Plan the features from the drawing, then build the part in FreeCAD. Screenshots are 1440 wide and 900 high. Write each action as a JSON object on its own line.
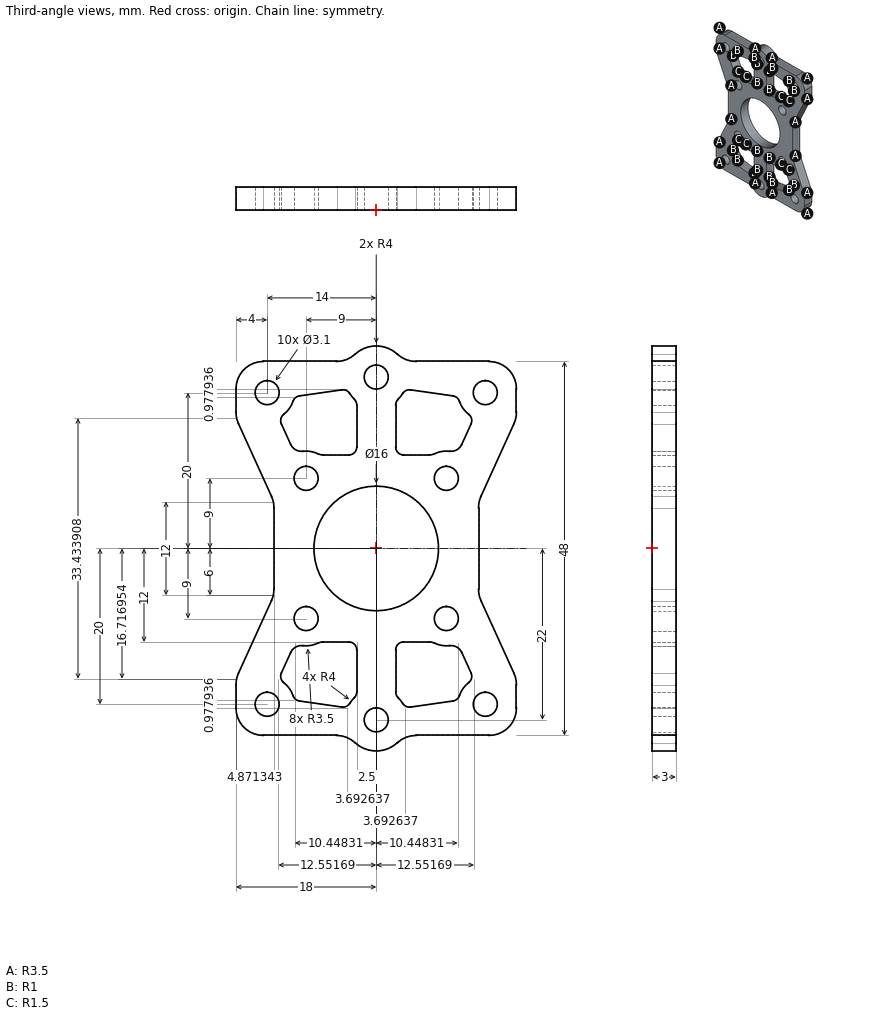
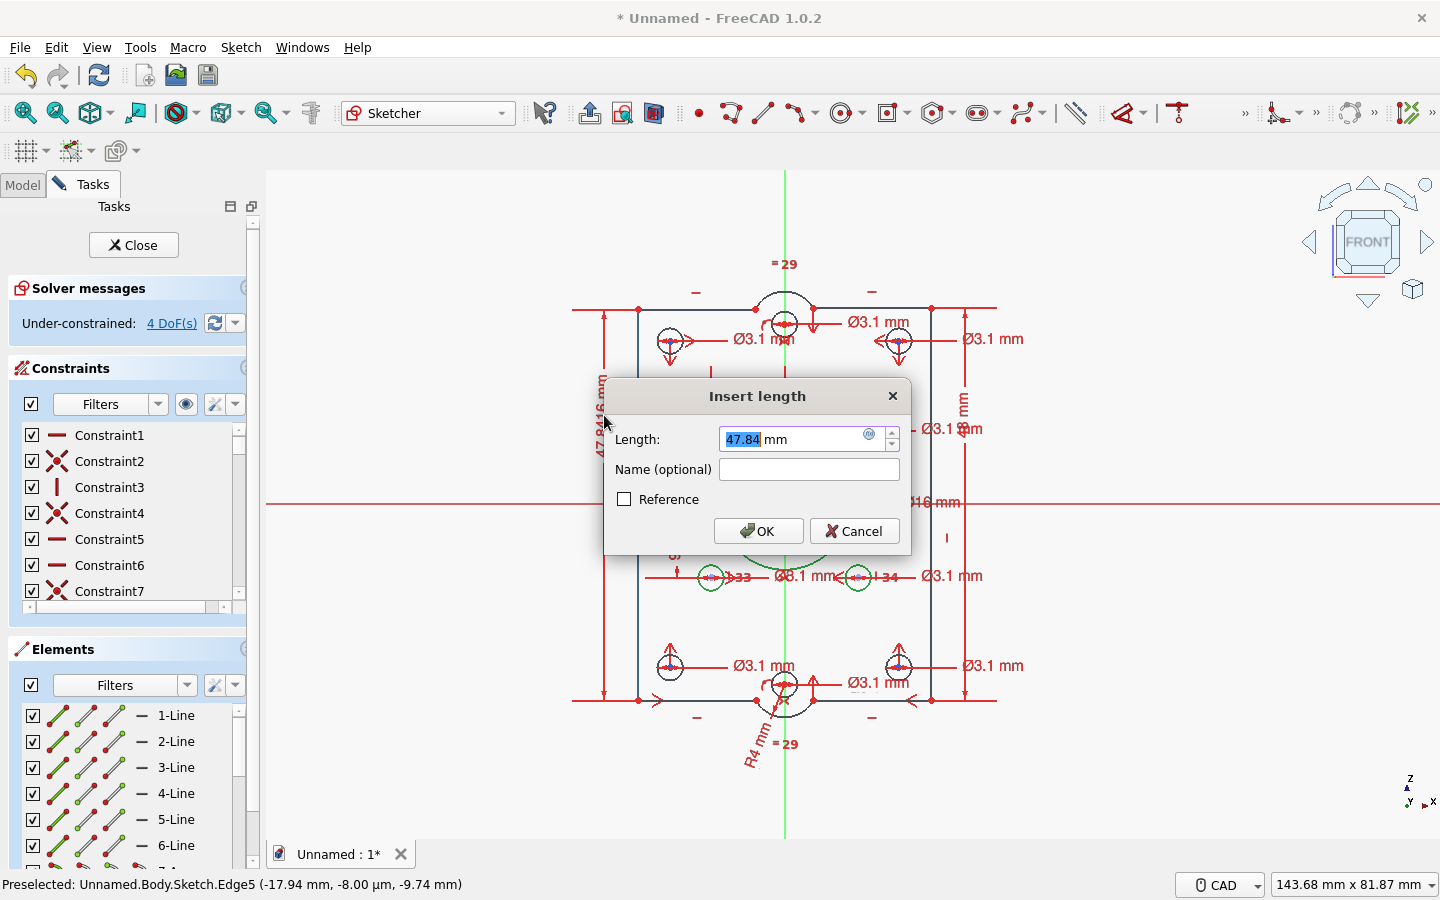
{"action": "type", "text": "48"}
{"action": "key", "text": "Return"}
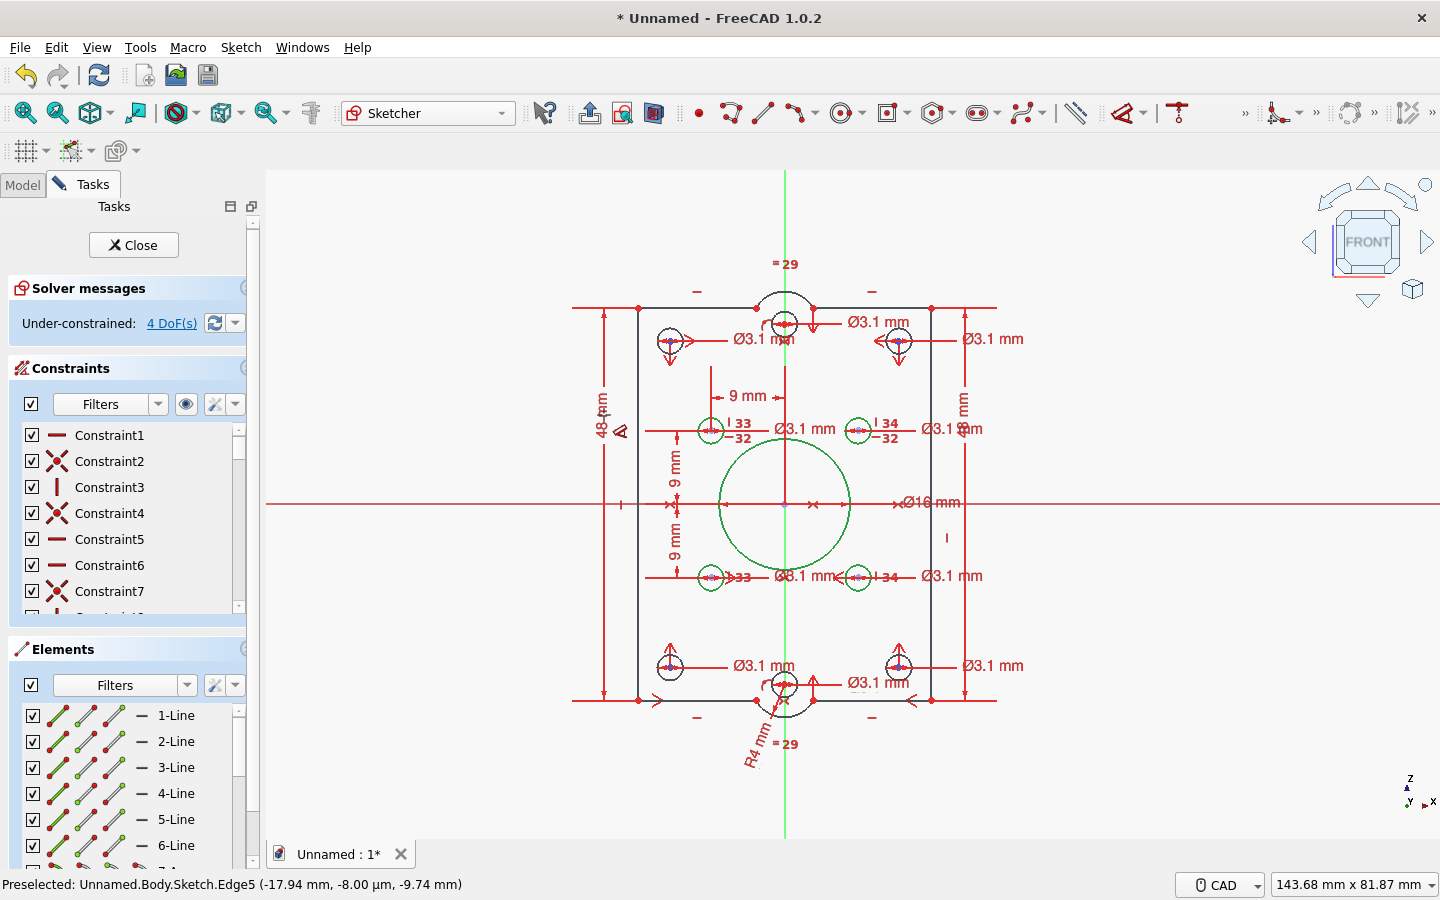
{"action": "left_click", "coordinate": [670, 341]}
{"action": "left_click", "coordinate": [754, 538]}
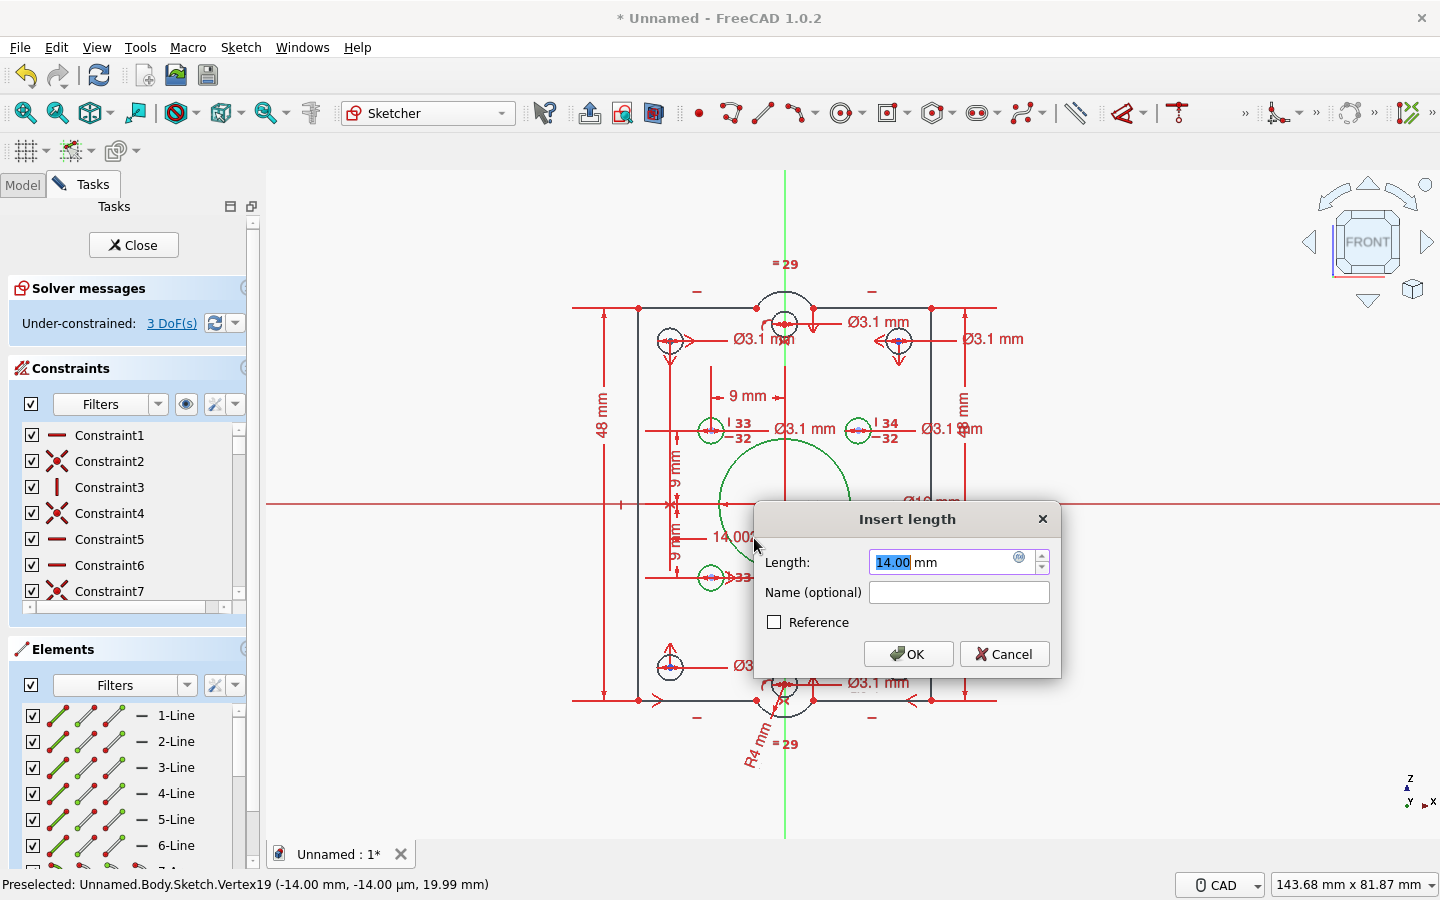
{"action": "type", "text": "14"}
{"action": "key", "text": "Return"}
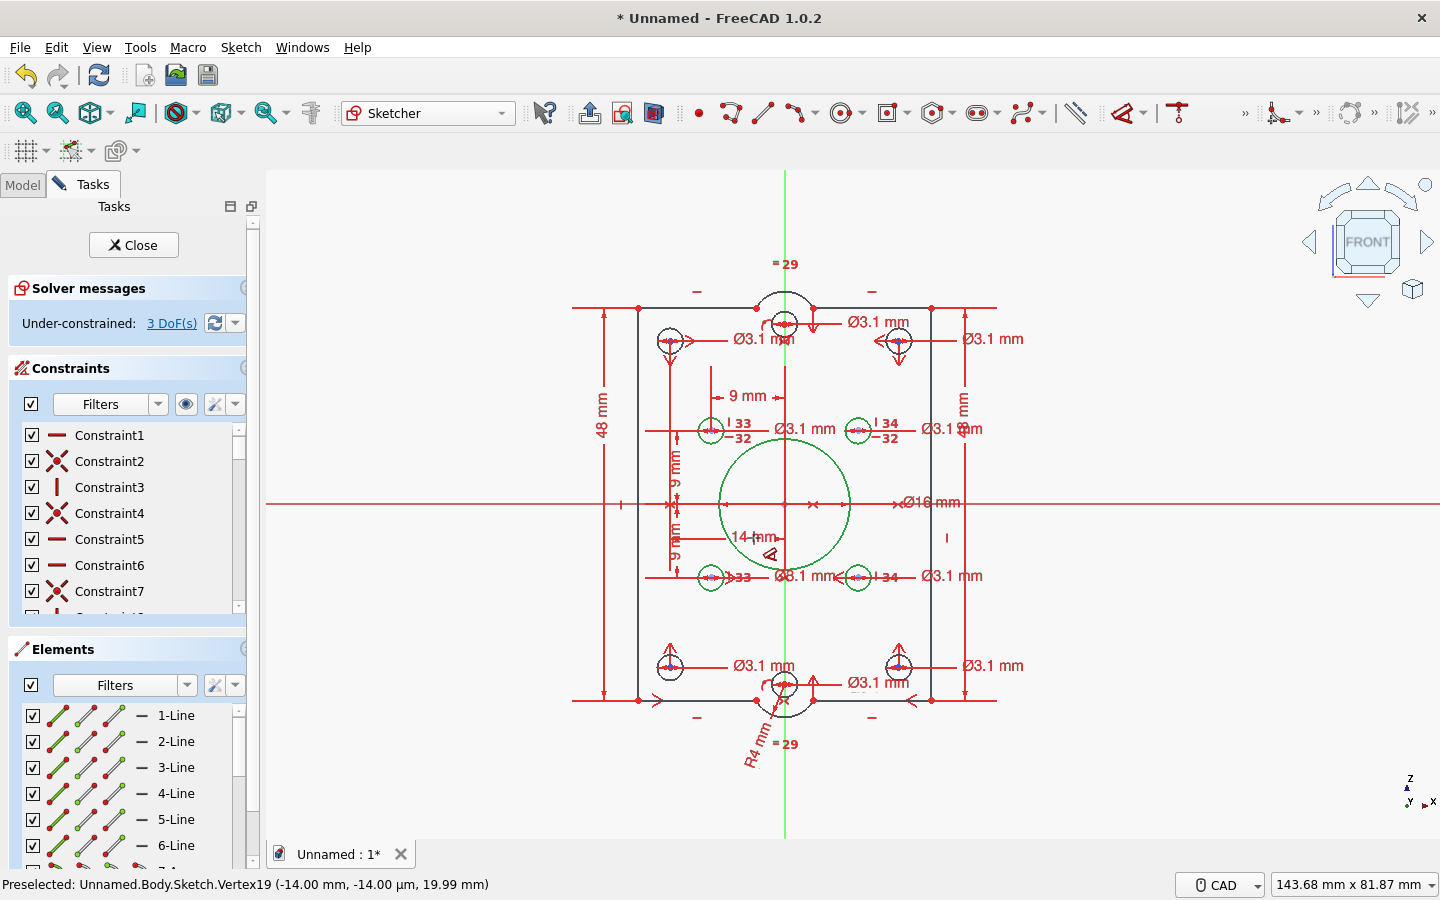
{"action": "left_click", "coordinate": [670, 341]}
{"action": "left_click", "coordinate": [819, 423]}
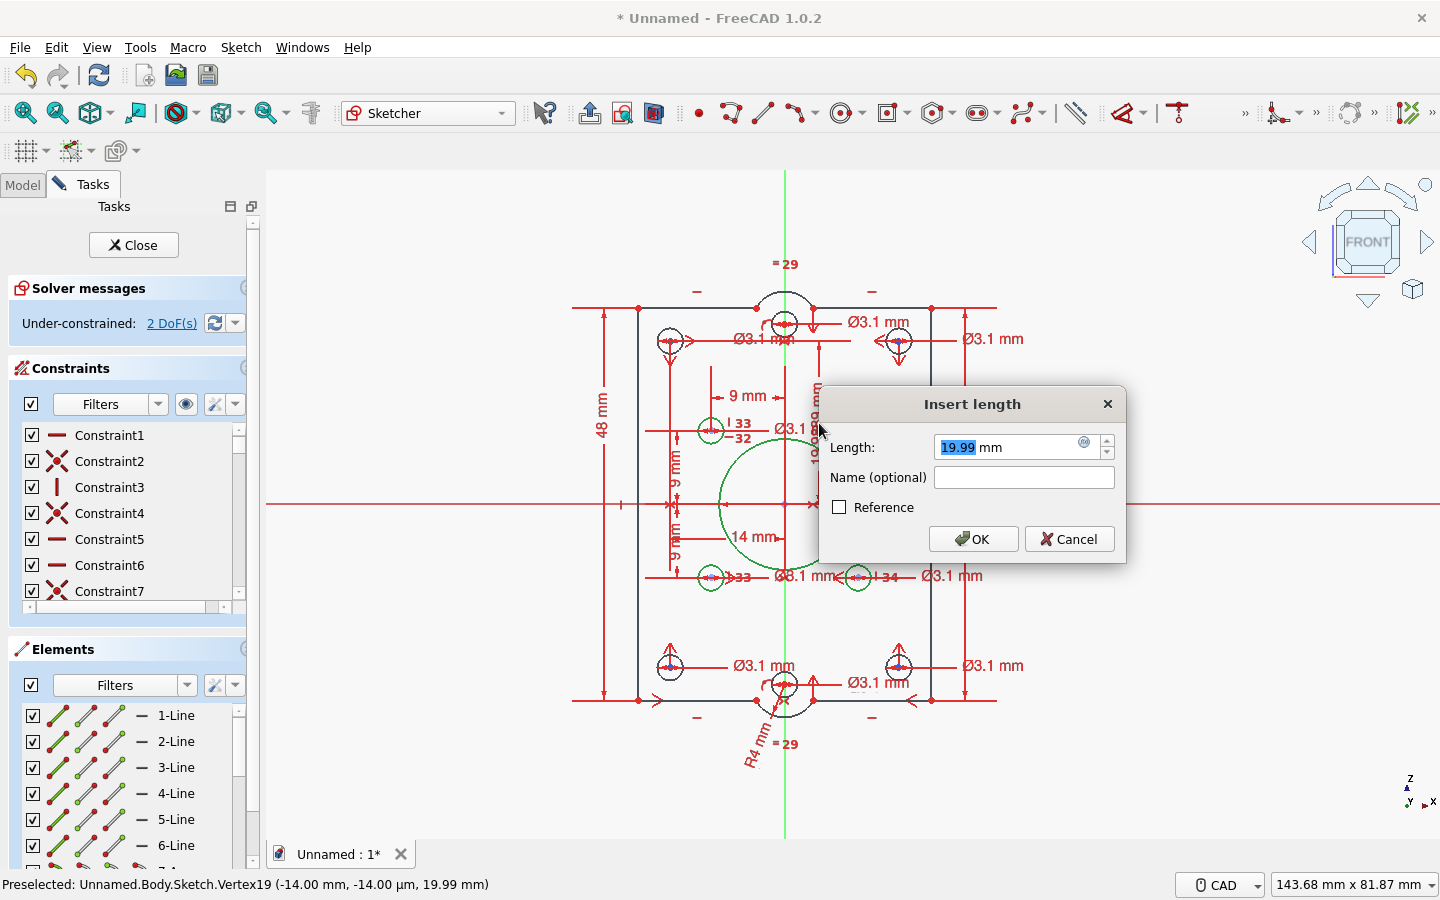
{"action": "type", "text": "20"}
{"action": "key", "text": "Return"}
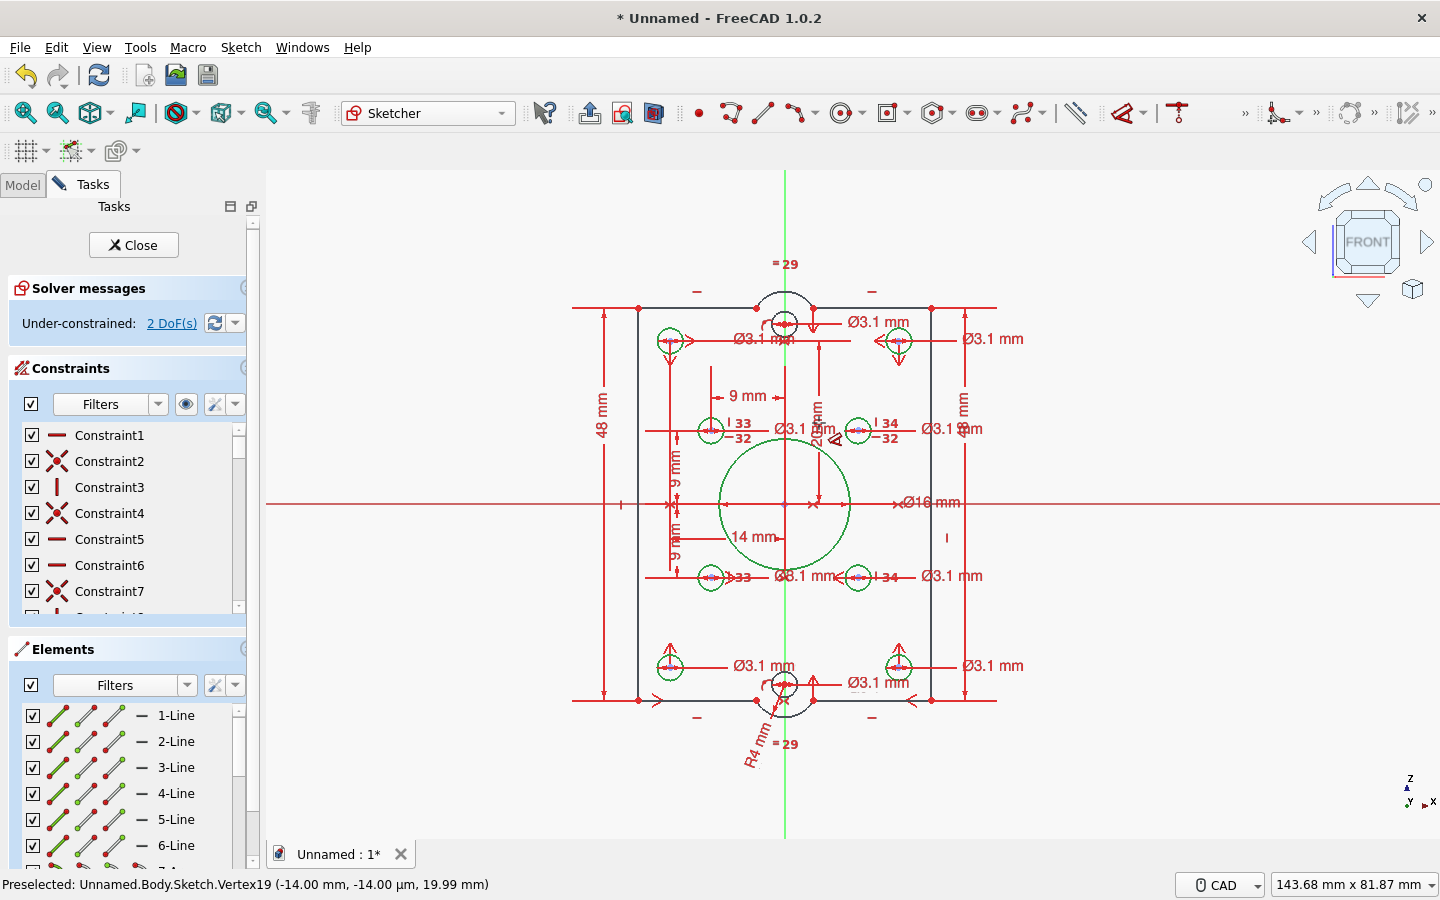
{"action": "left_click", "coordinate": [785, 685]}
{"action": "left_click", "coordinate": [819, 595]}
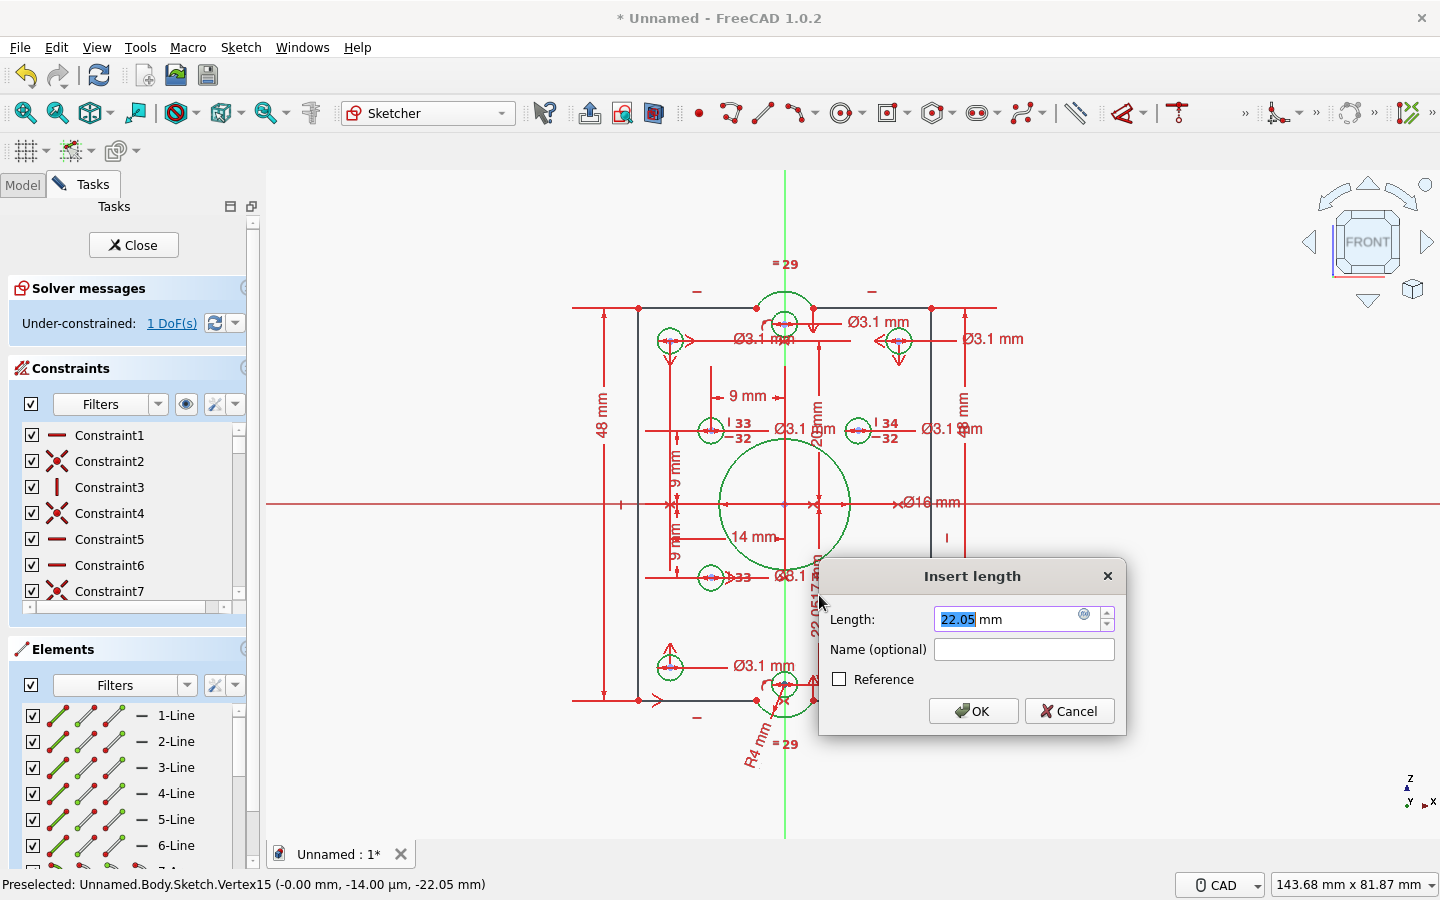
{"action": "type", "text": "22"}
{"action": "key", "text": "Return"}